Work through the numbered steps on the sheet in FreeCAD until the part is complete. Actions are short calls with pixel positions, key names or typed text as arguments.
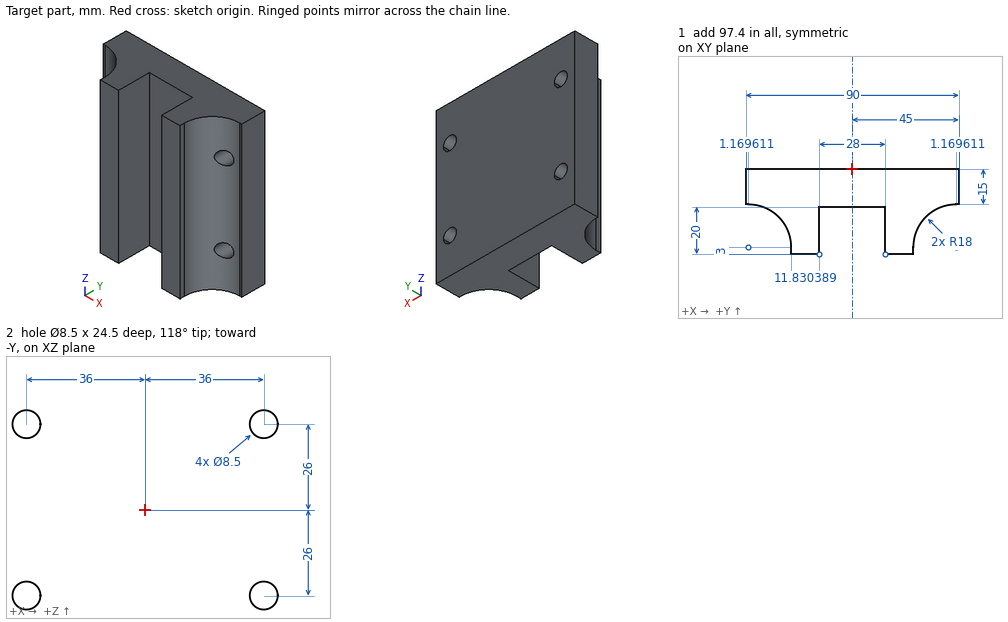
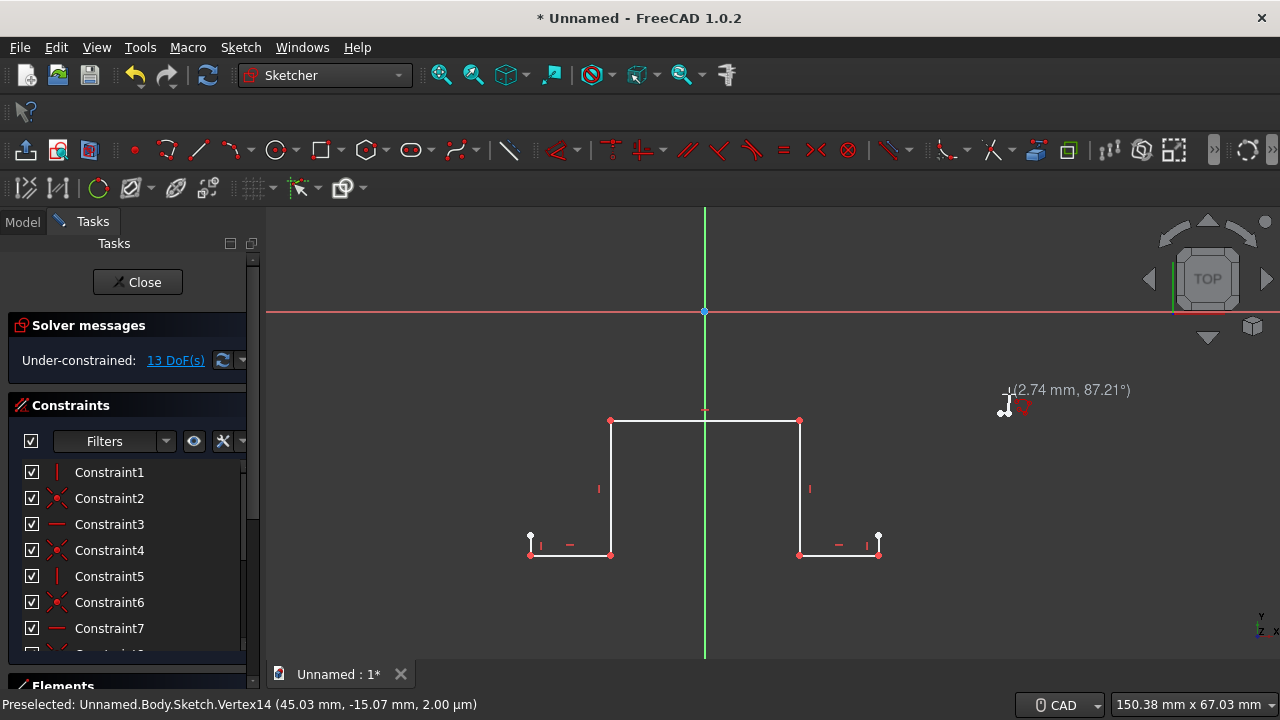
click(1009, 312)
click(401, 321)
click(401, 413)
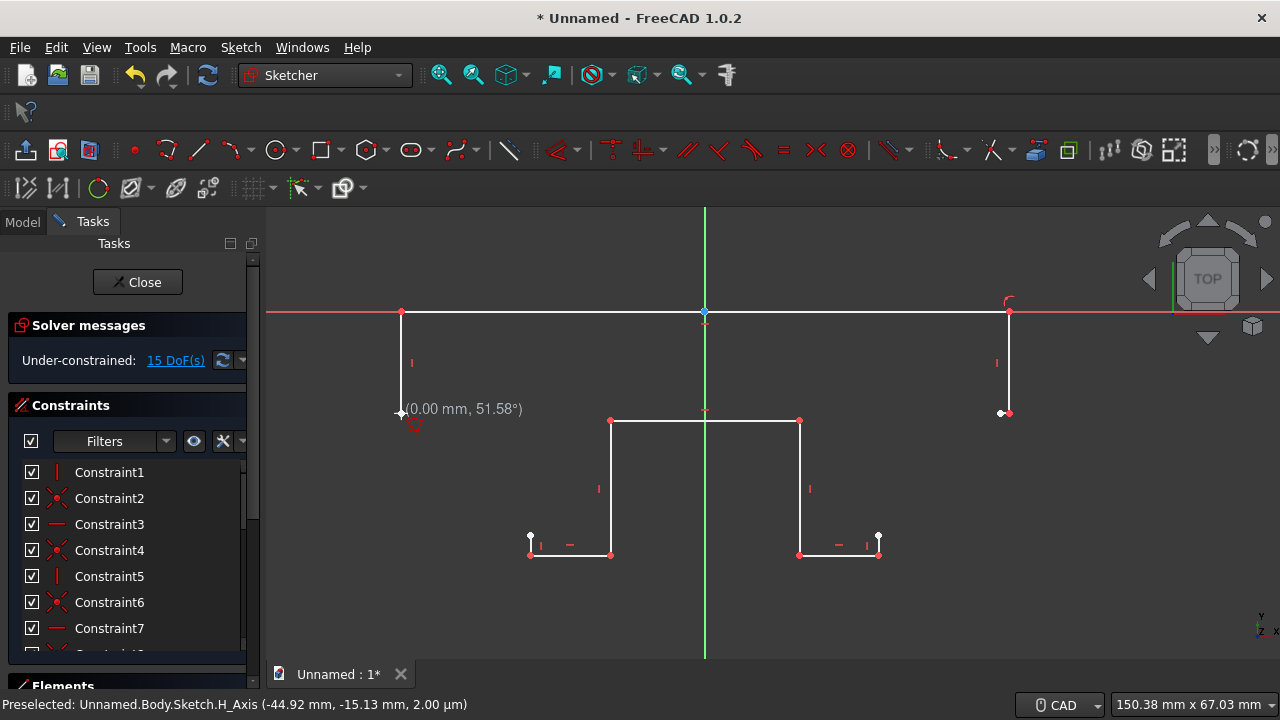
scroll(409, 413, up, 4)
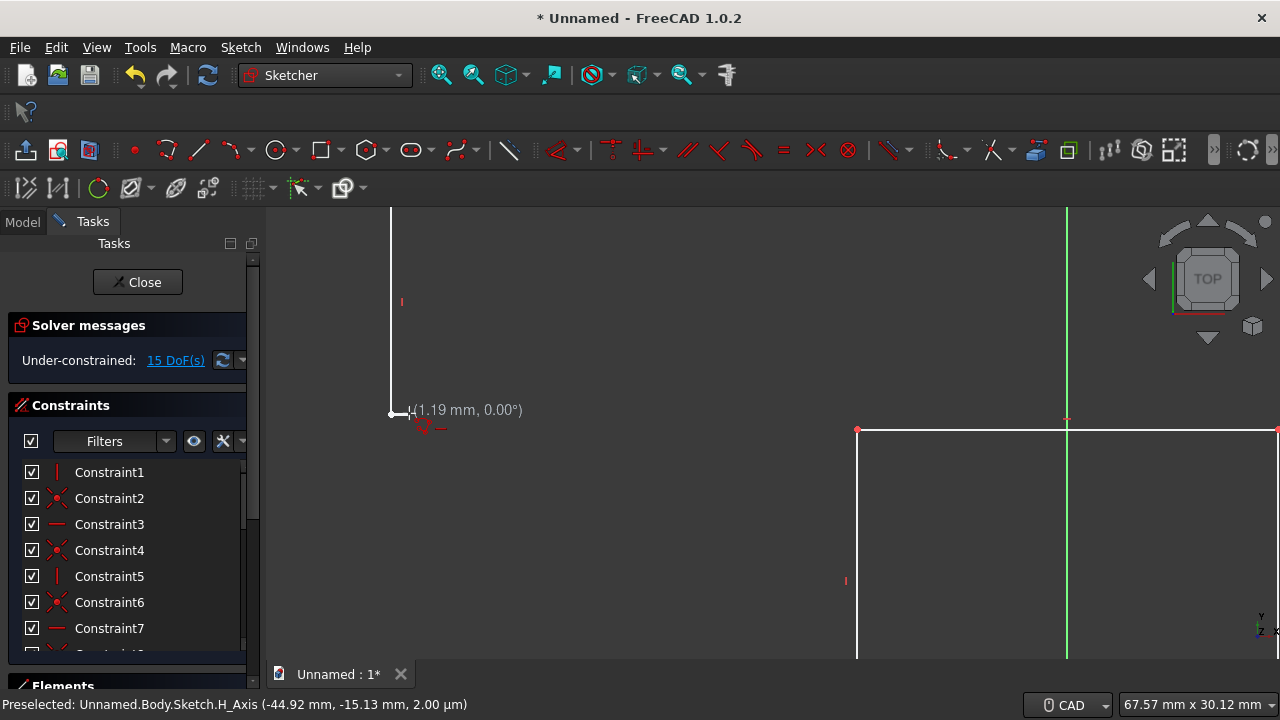
click(410, 412)
right_click(410, 412)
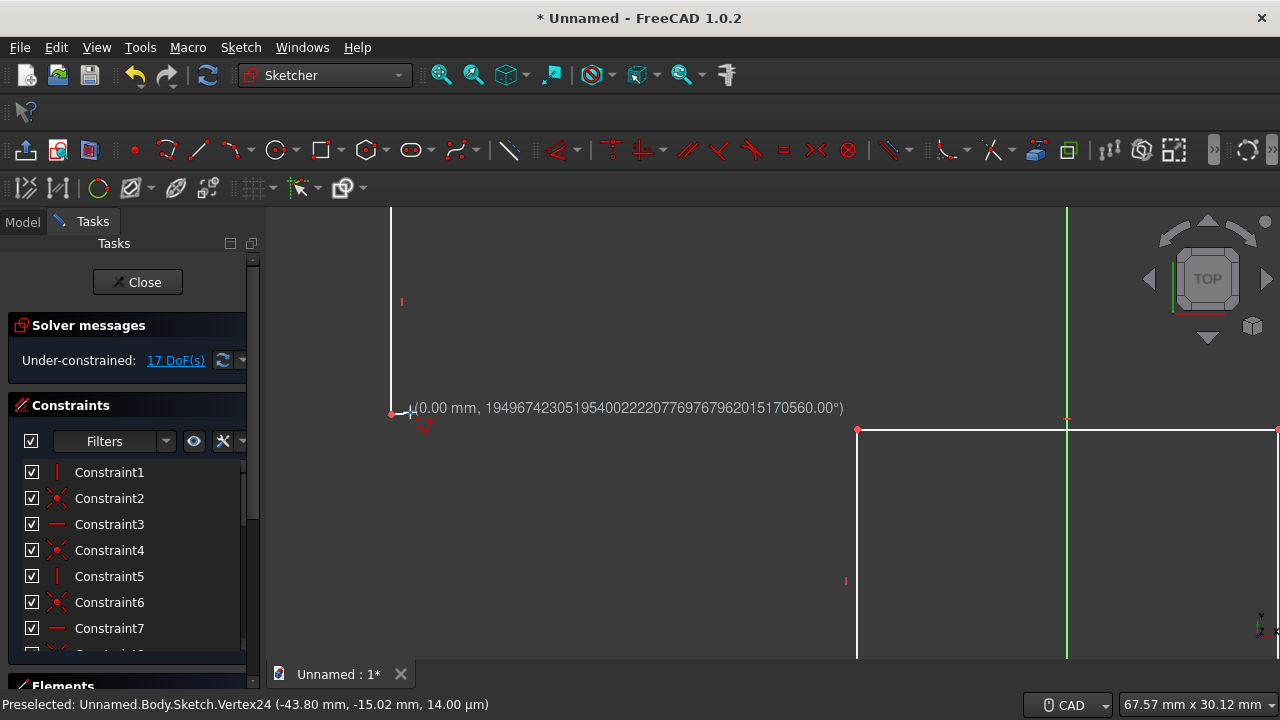
click(232, 150)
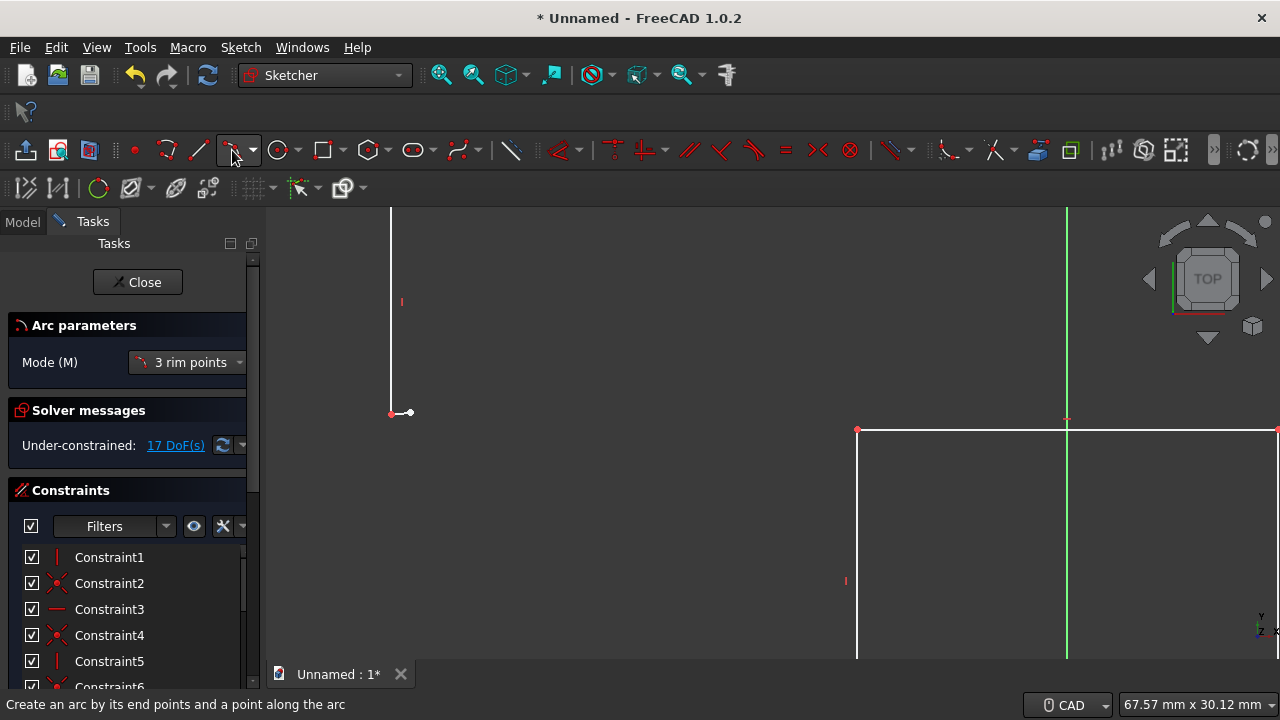
scroll(408, 413, down, 4)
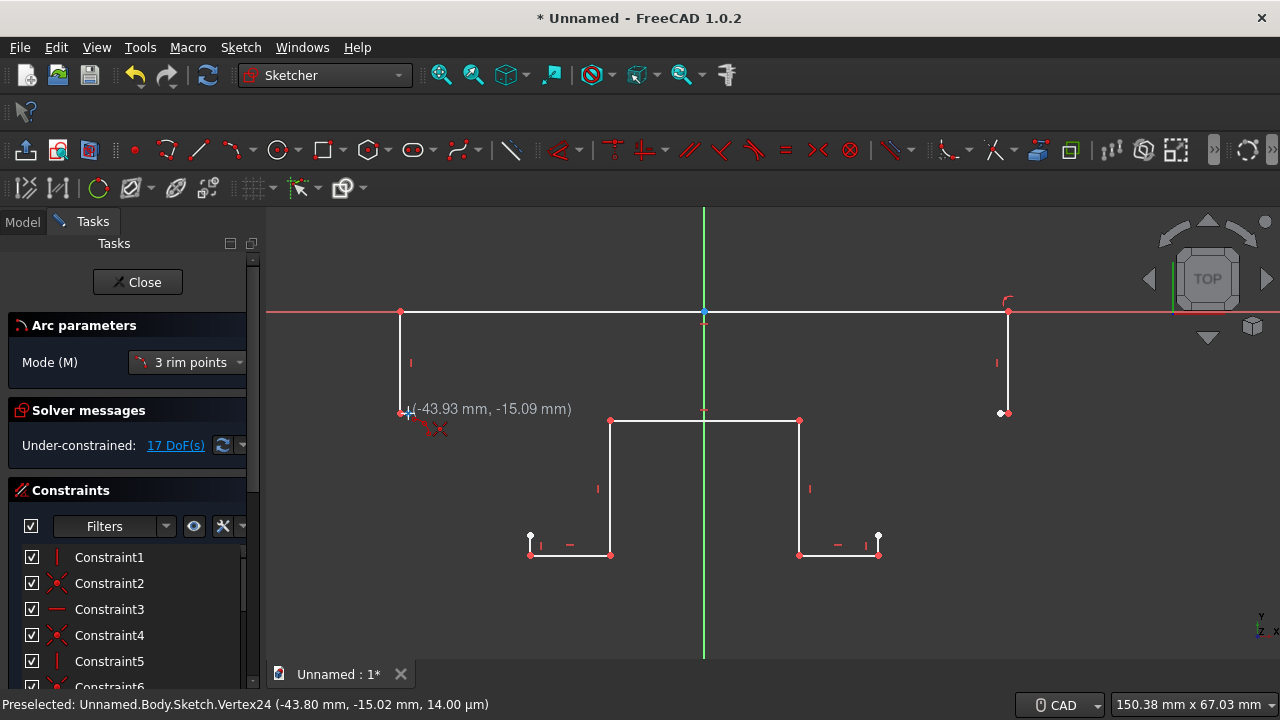
scroll(878, 534, up, 3)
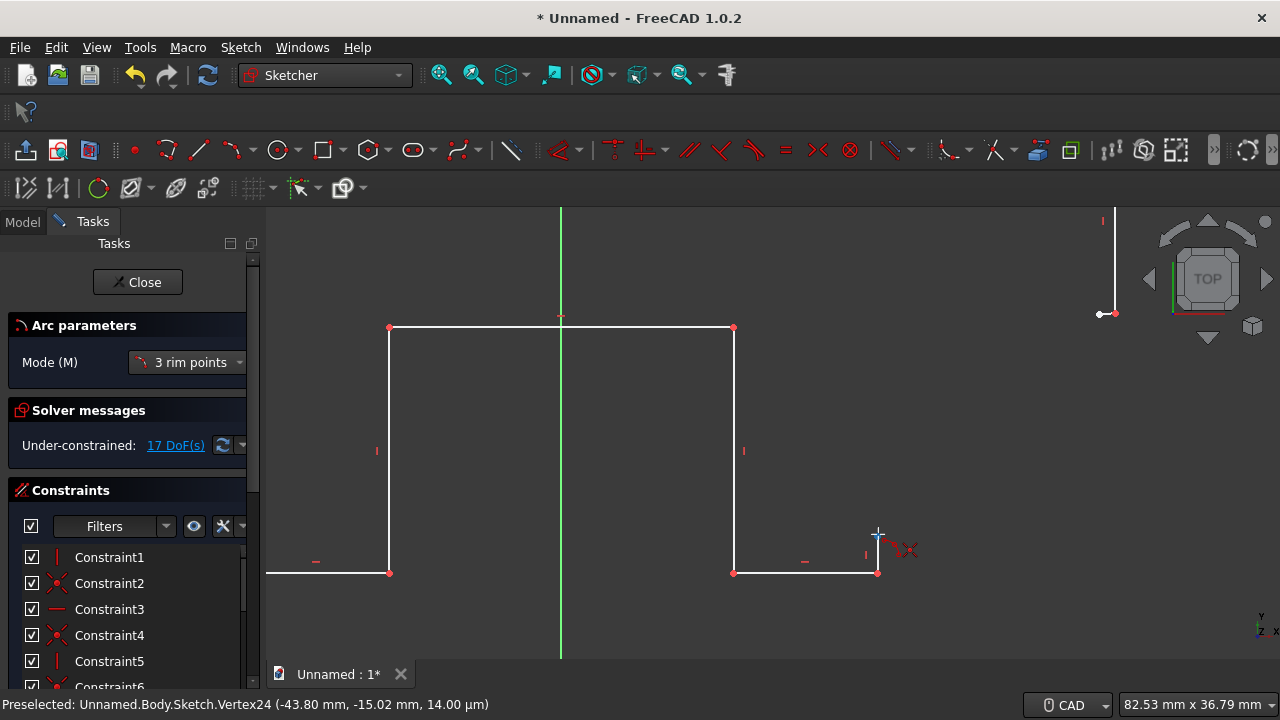
click(878, 537)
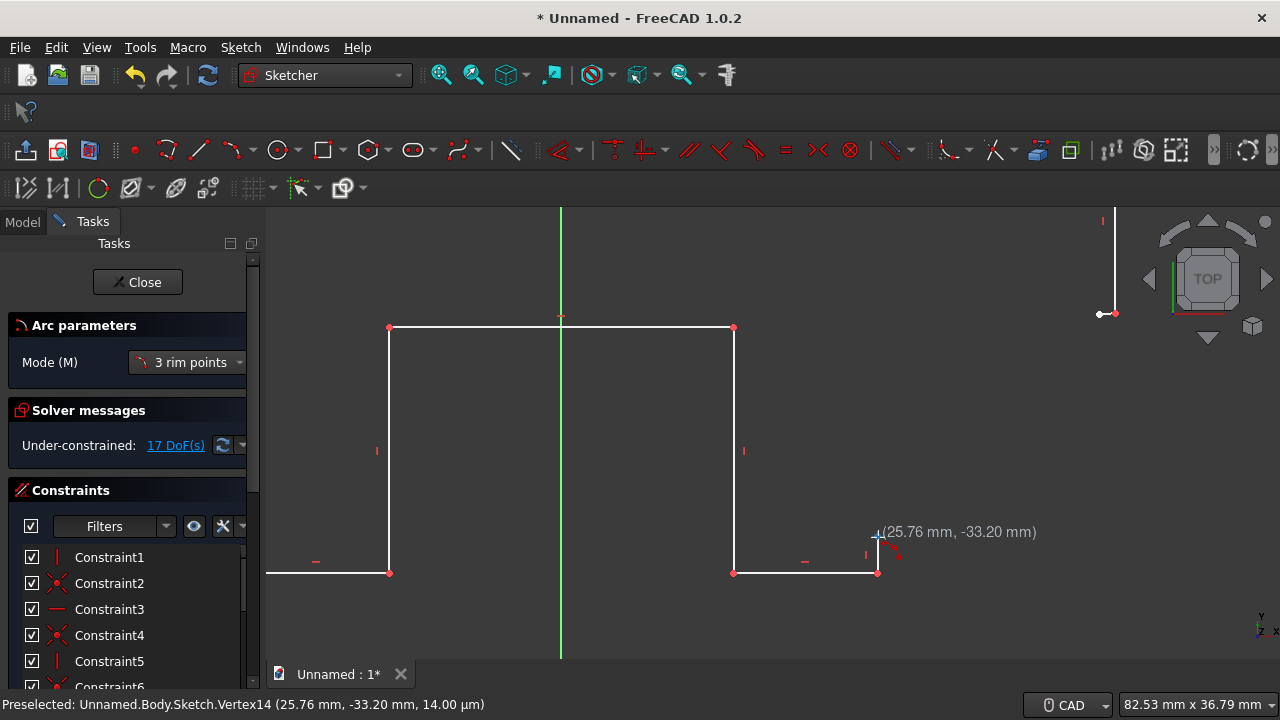
scroll(1100, 313, up, 4)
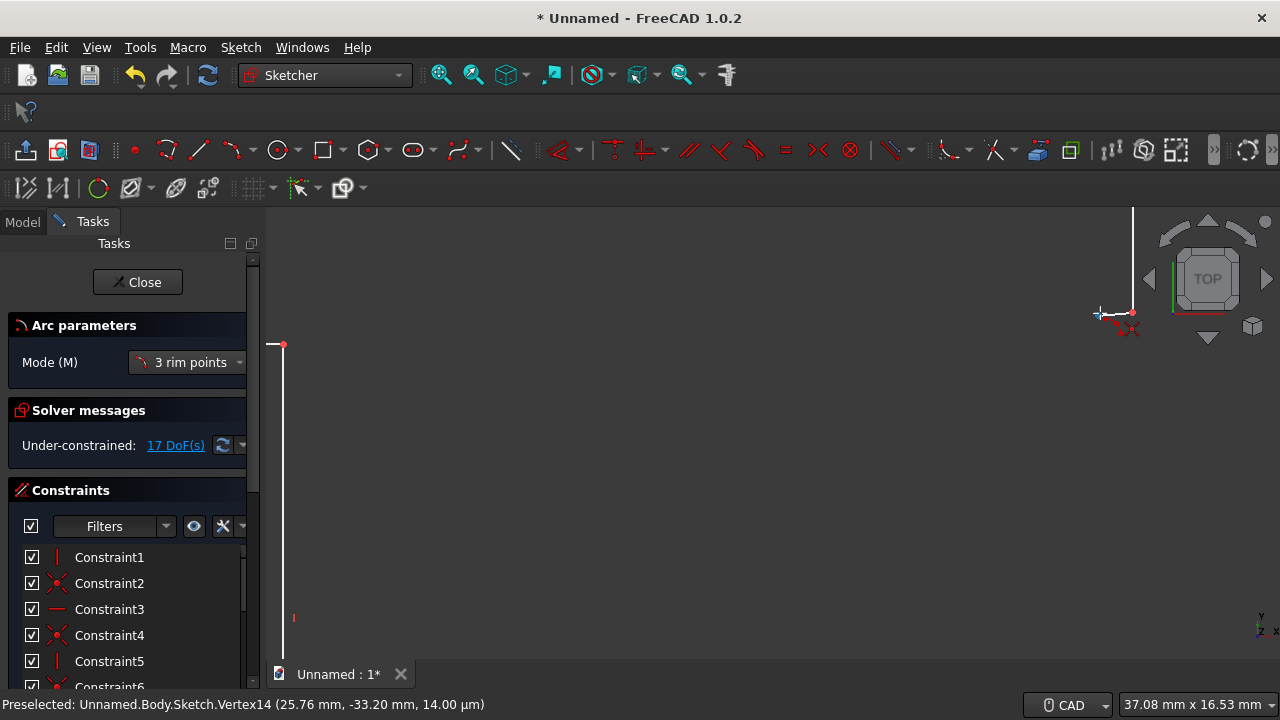
click(1099, 316)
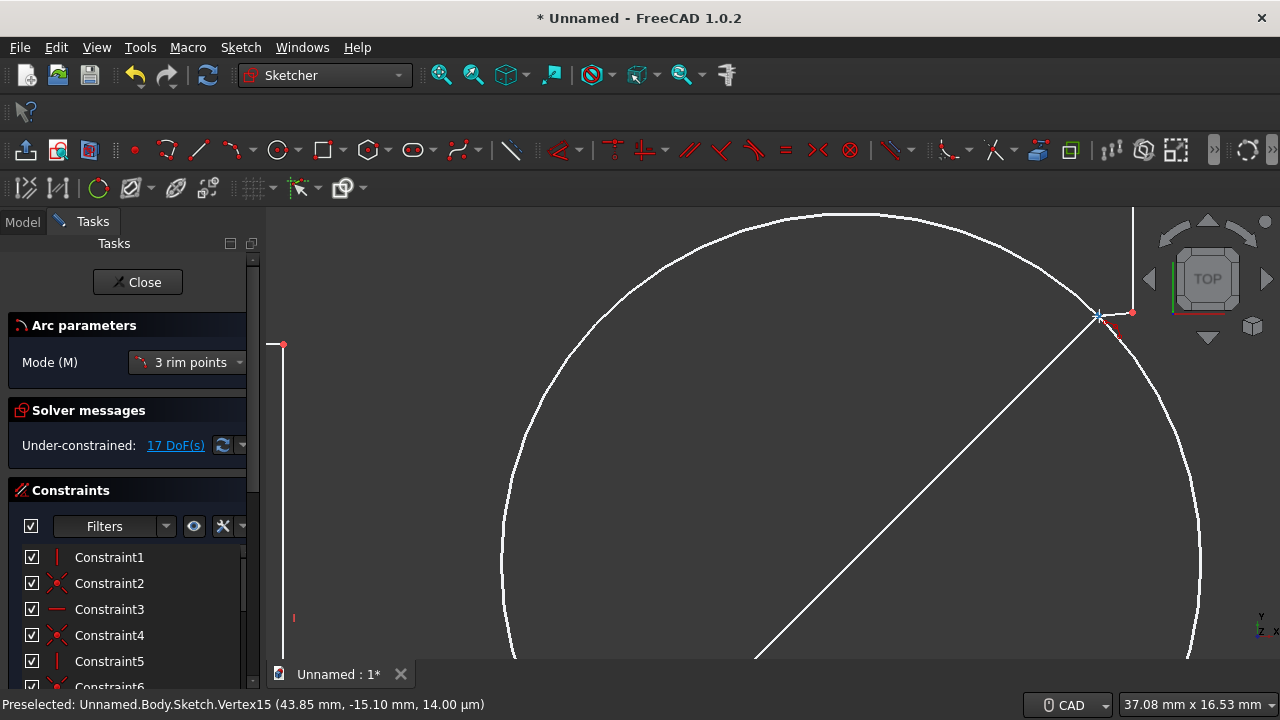
scroll(968, 445, down, 7)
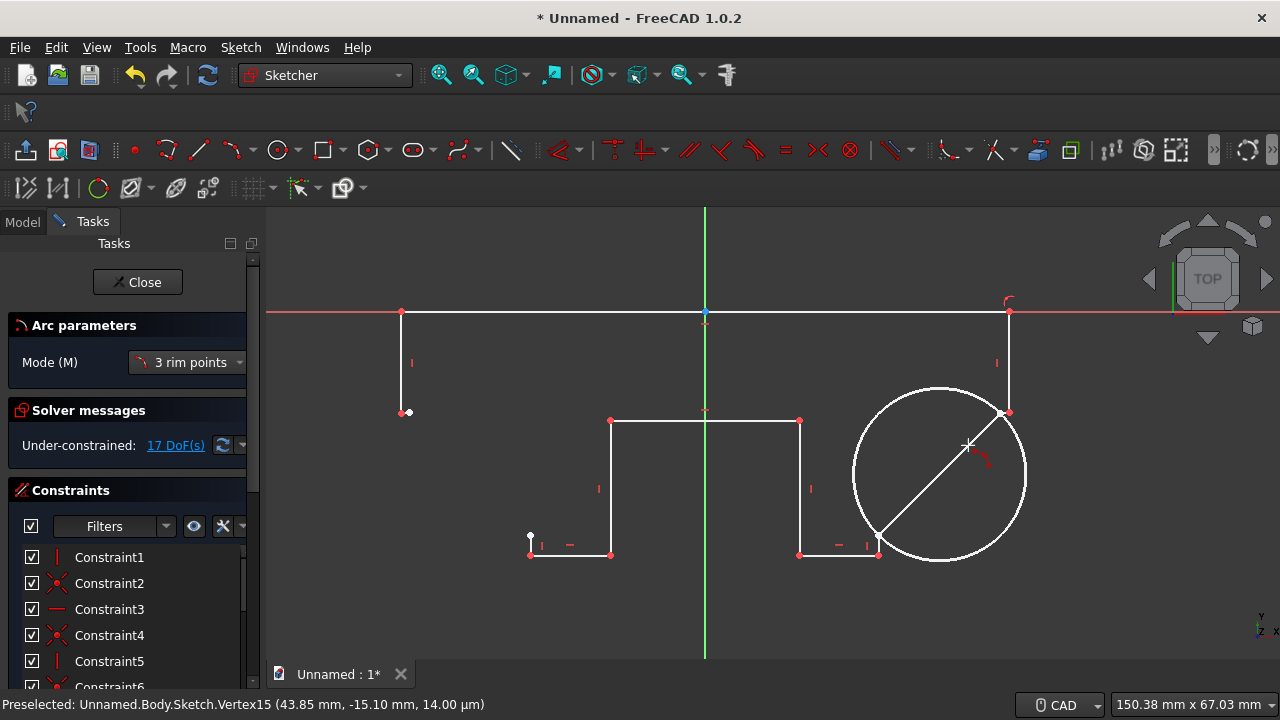
click(915, 448)